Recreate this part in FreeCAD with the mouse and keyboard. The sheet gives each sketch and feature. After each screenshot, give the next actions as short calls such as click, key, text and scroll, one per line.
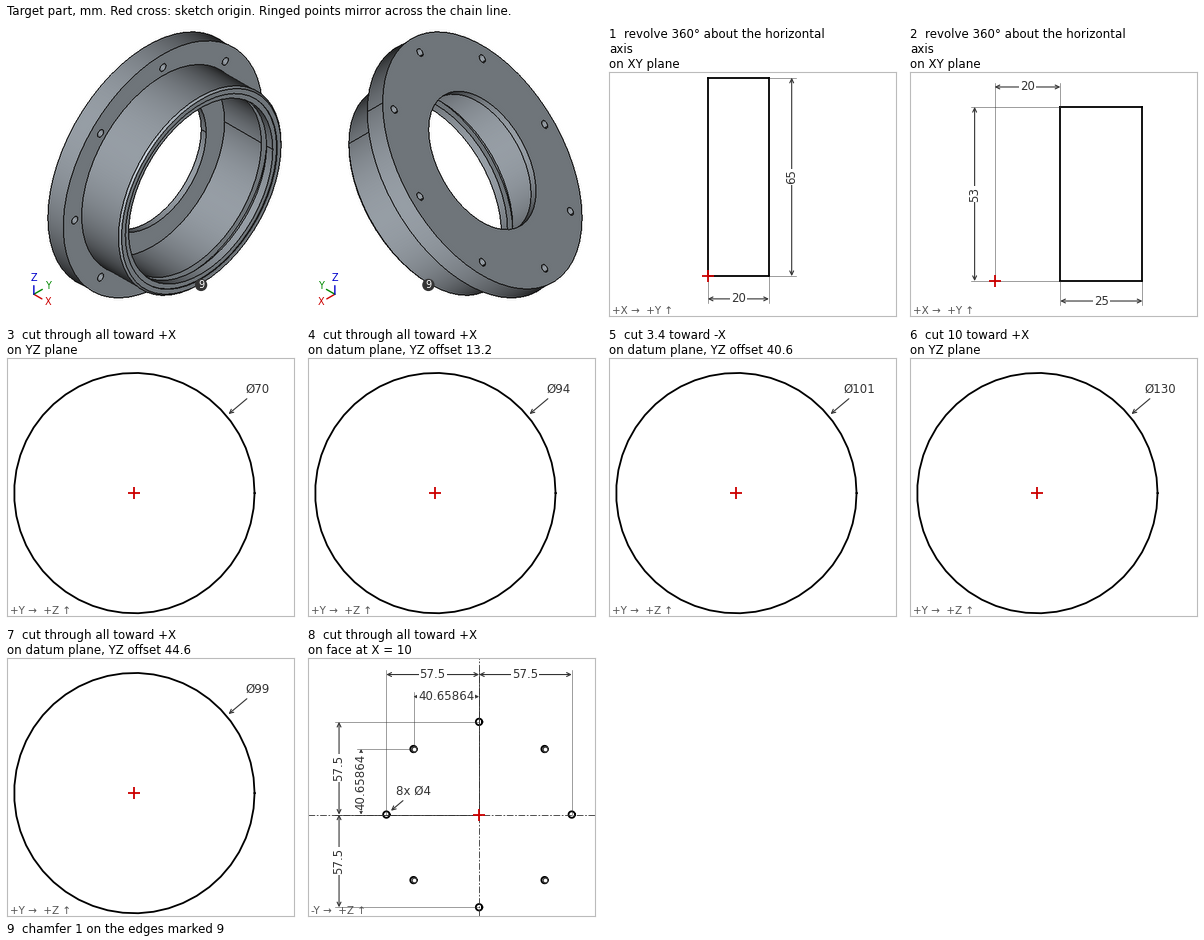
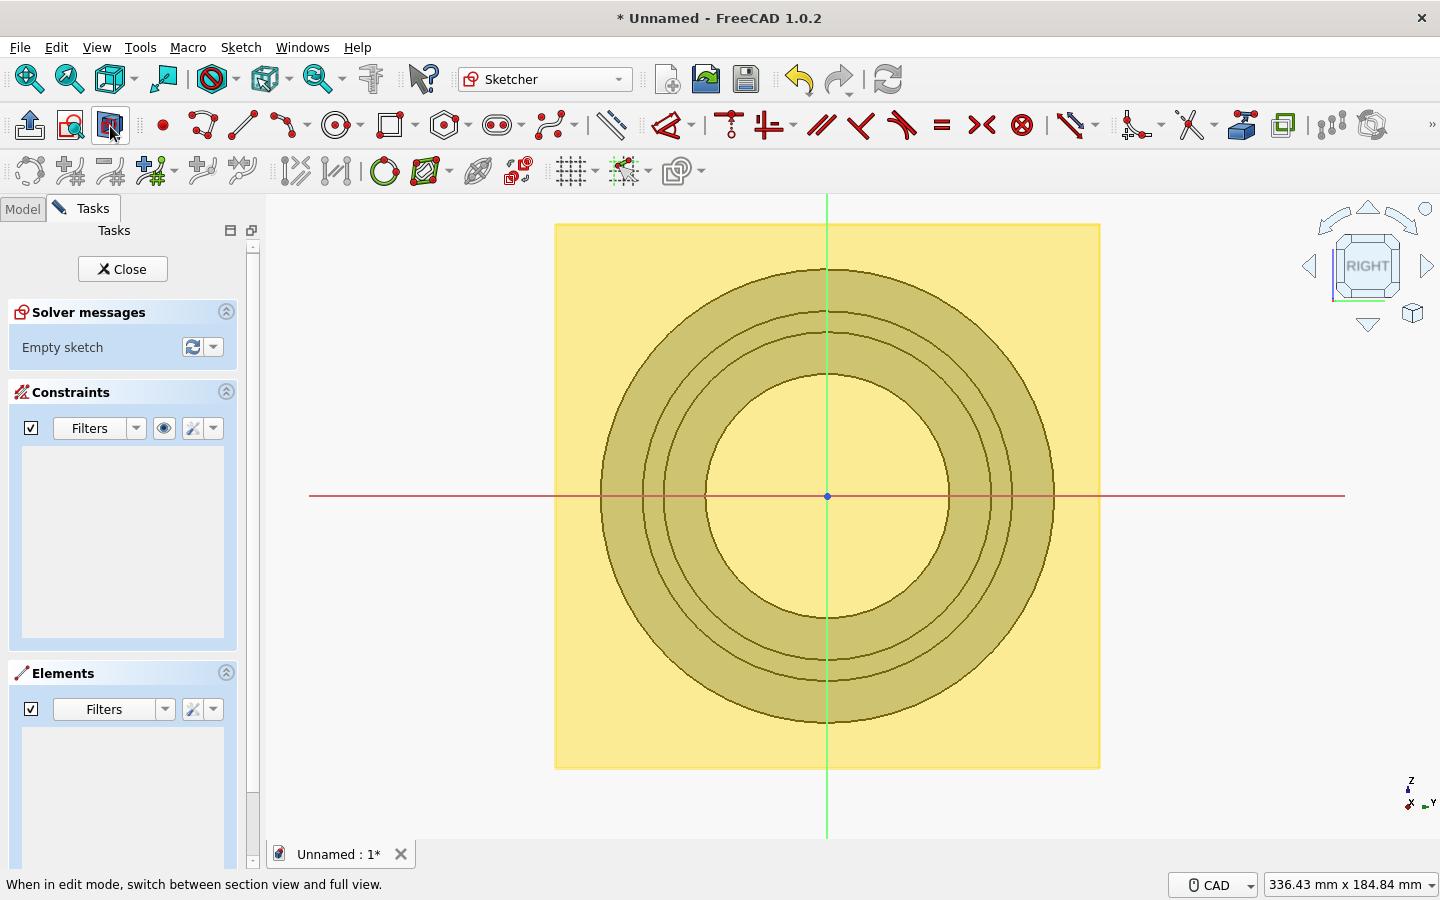
click(336, 126)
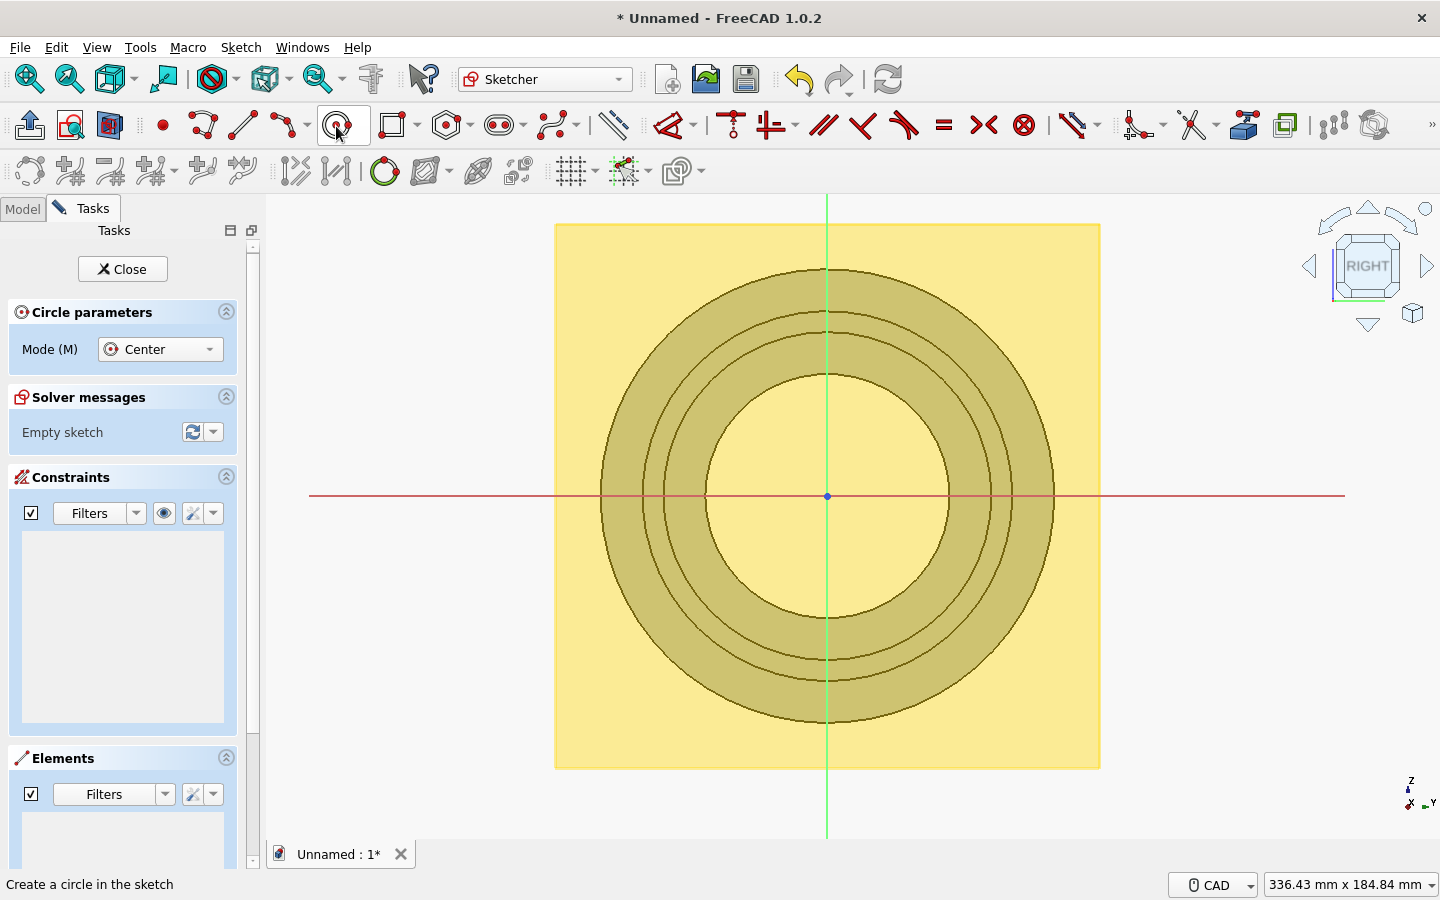
click(827, 496)
click(952, 372)
key(Escape)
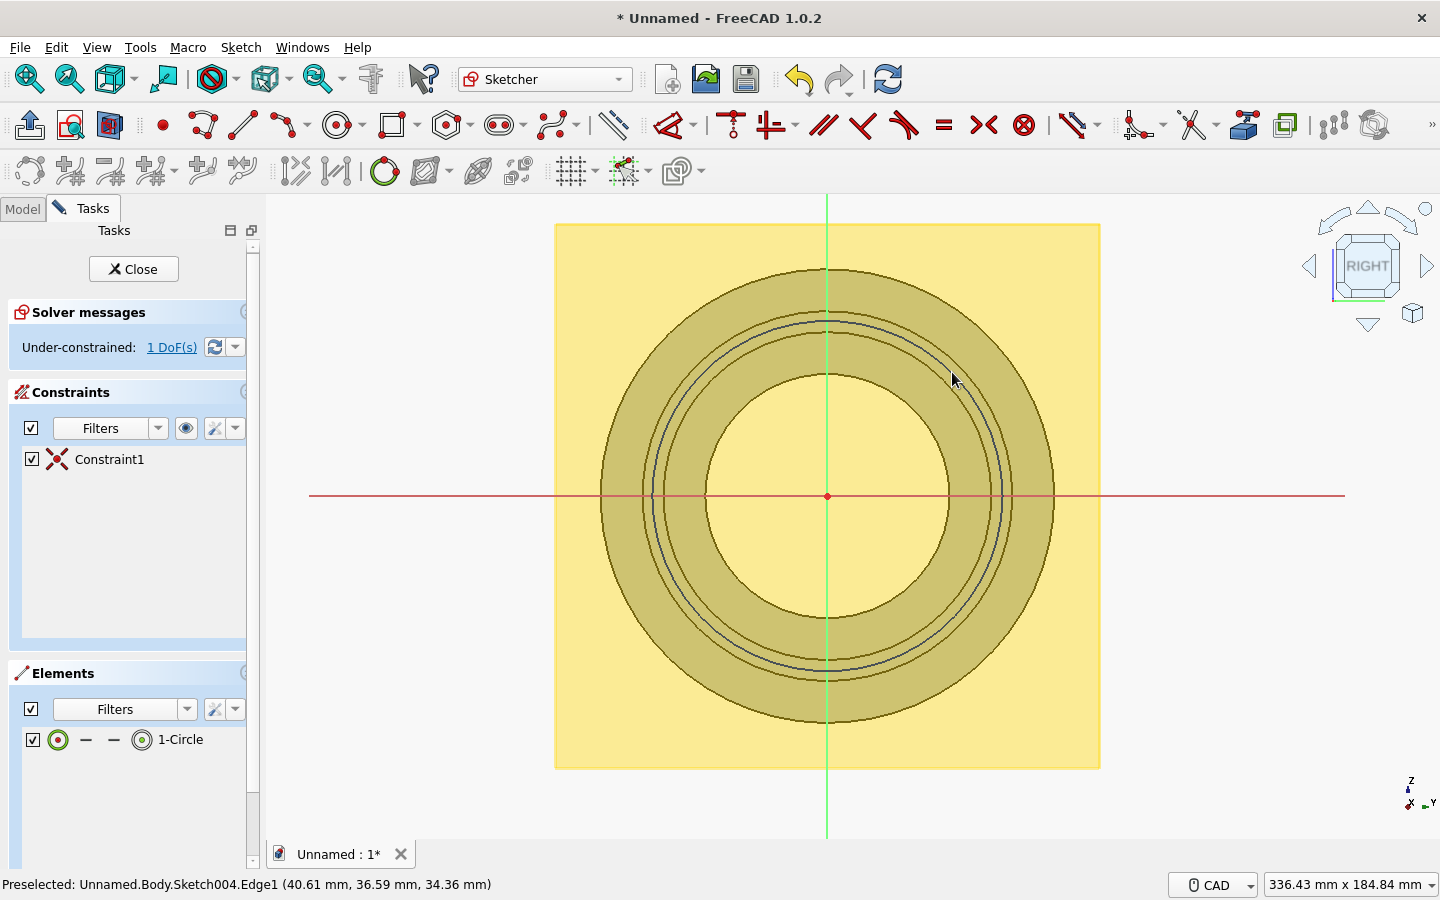
click(668, 126)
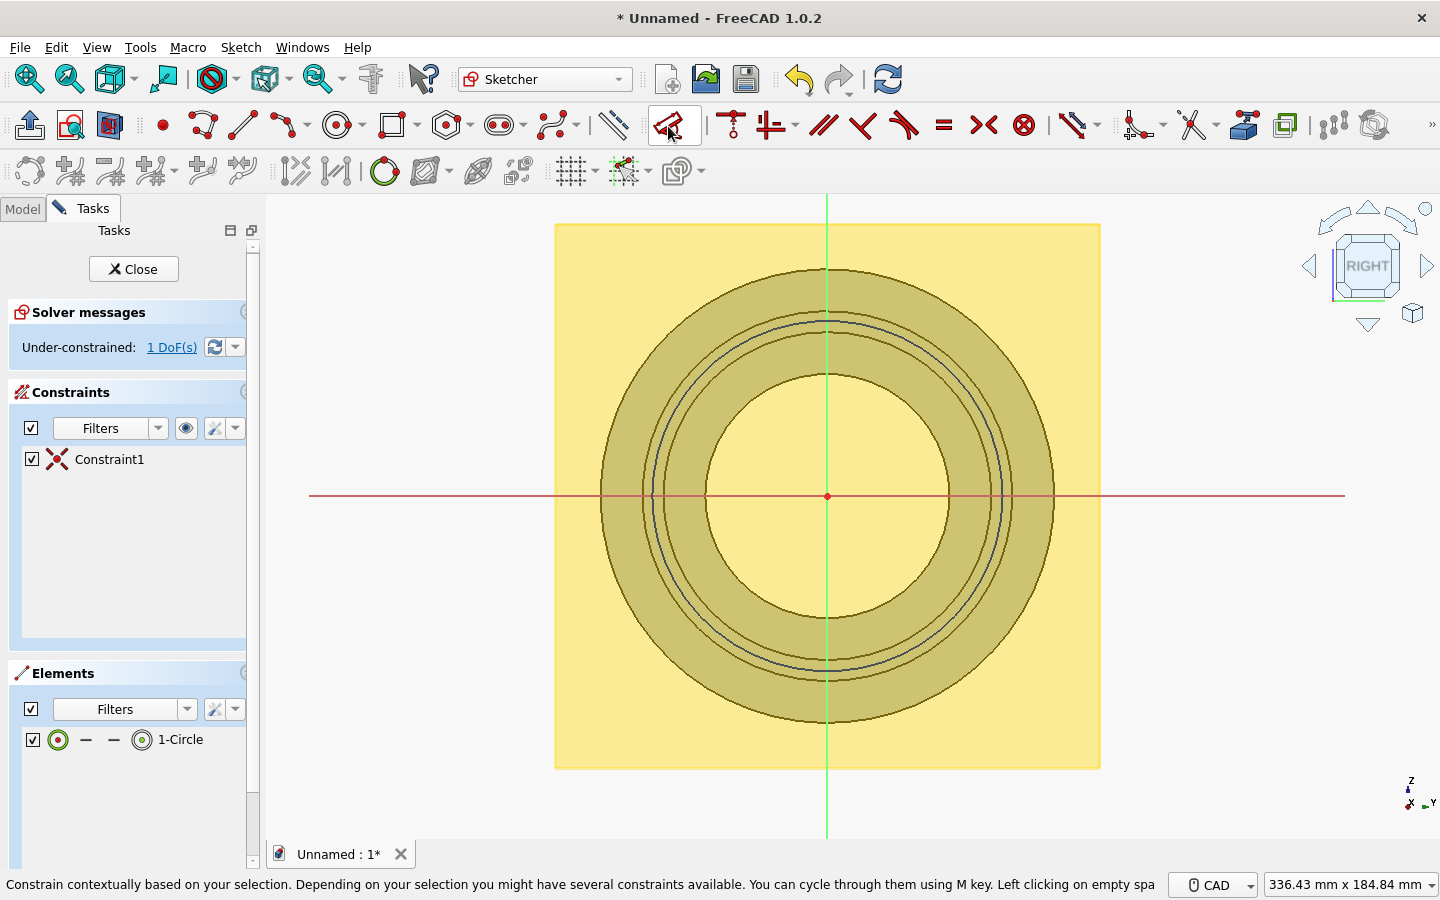
click(951, 372)
click(974, 349)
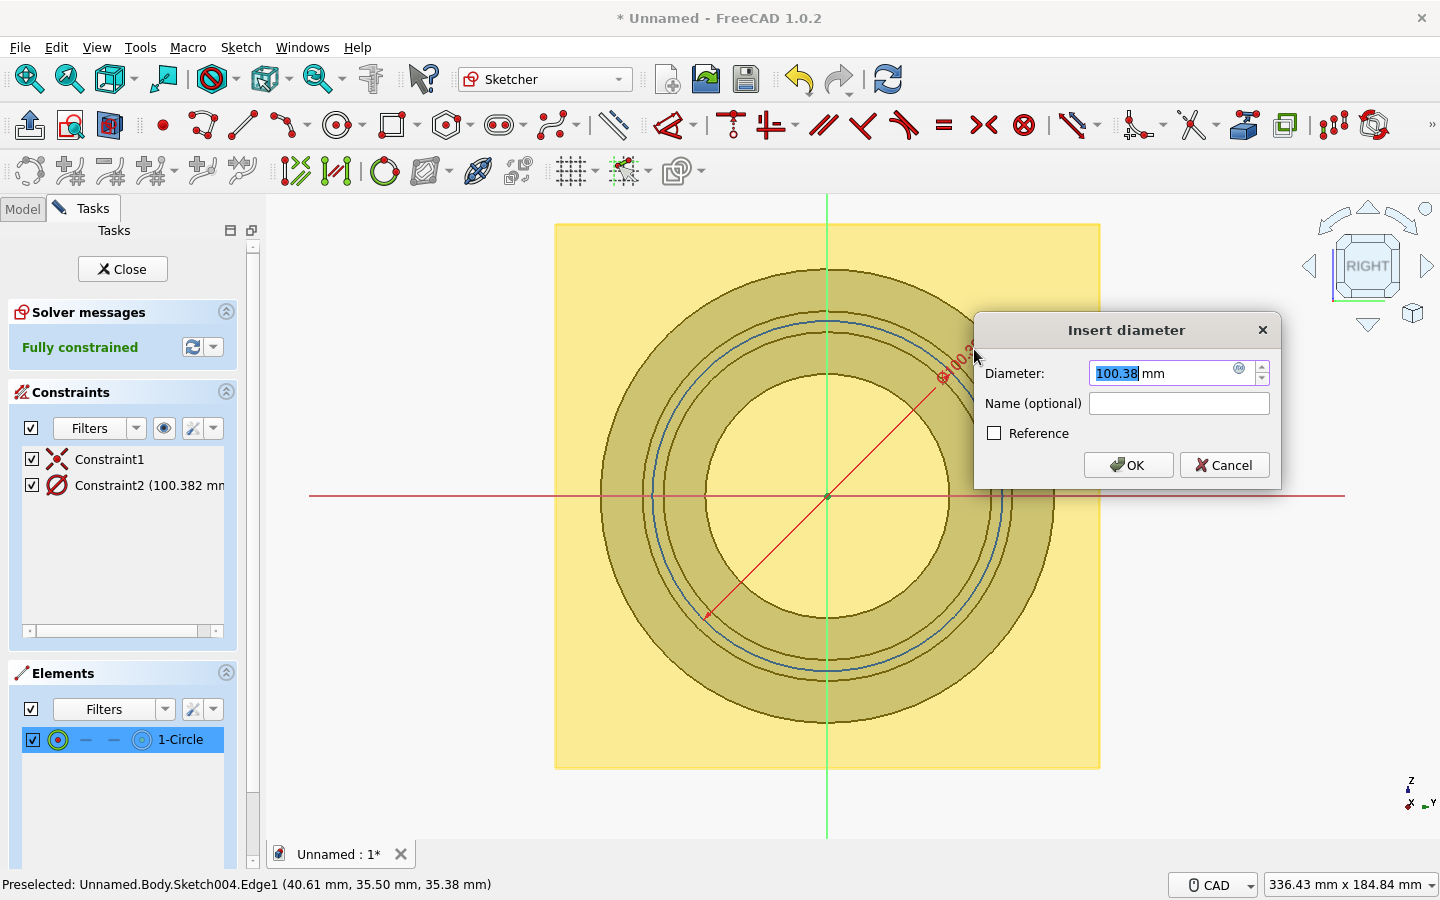
text(101)
key(Return)
key(Escape)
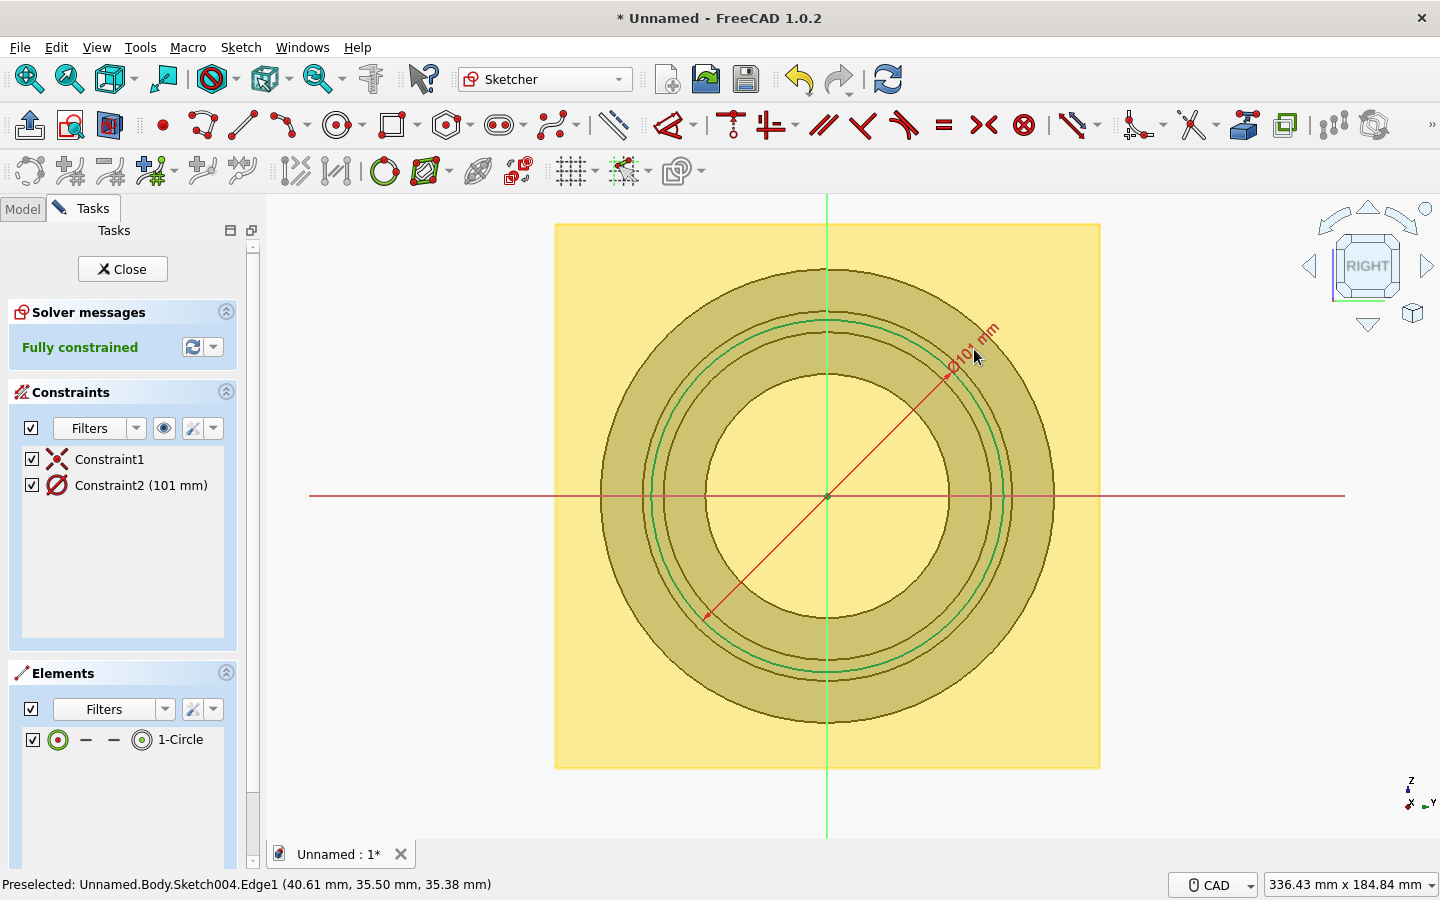
click(123, 269)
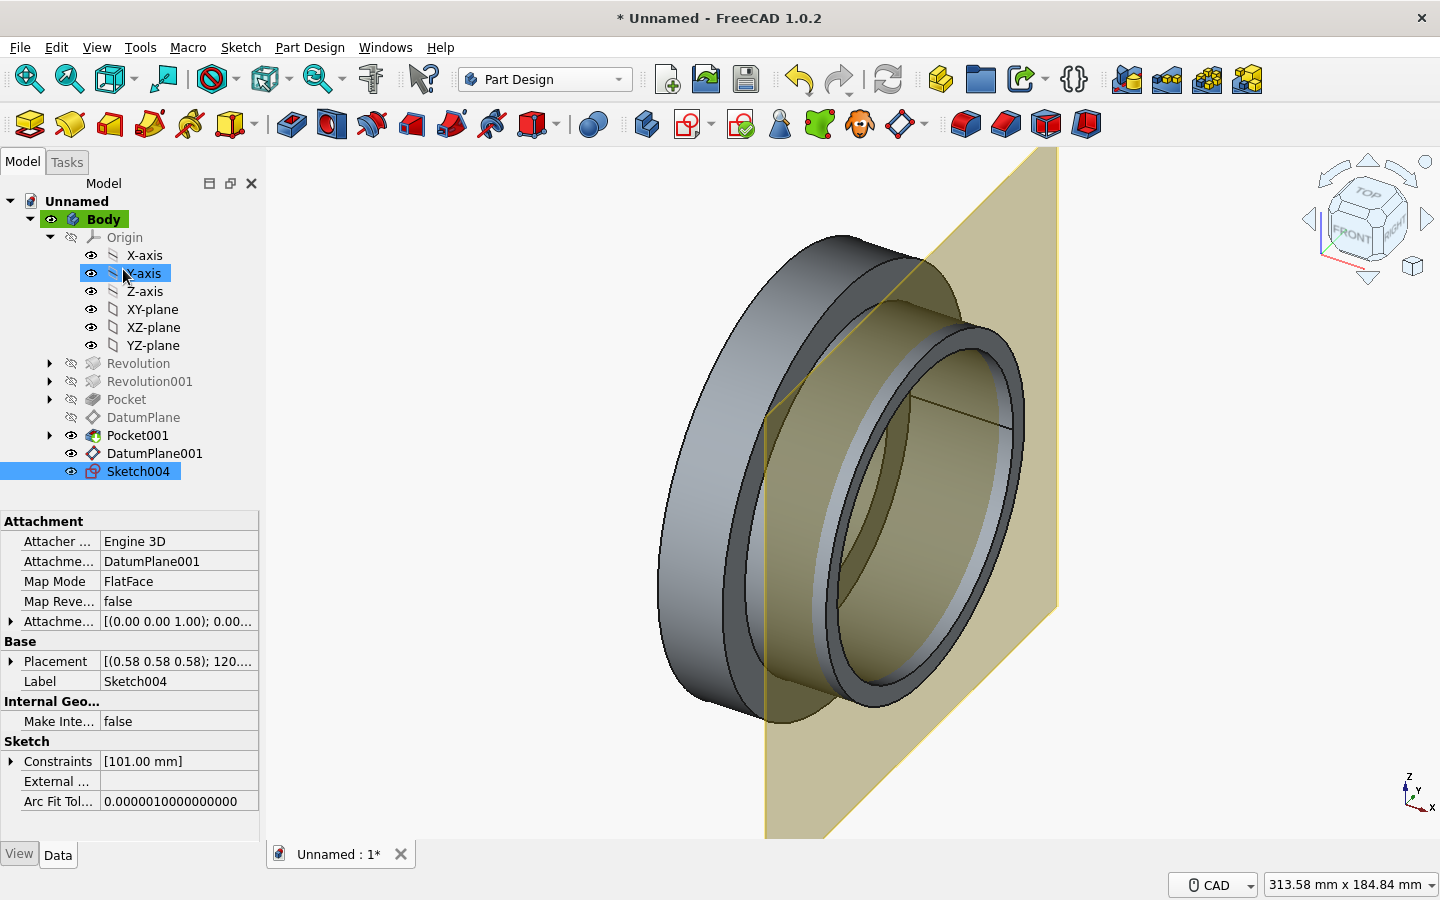
click(292, 124)